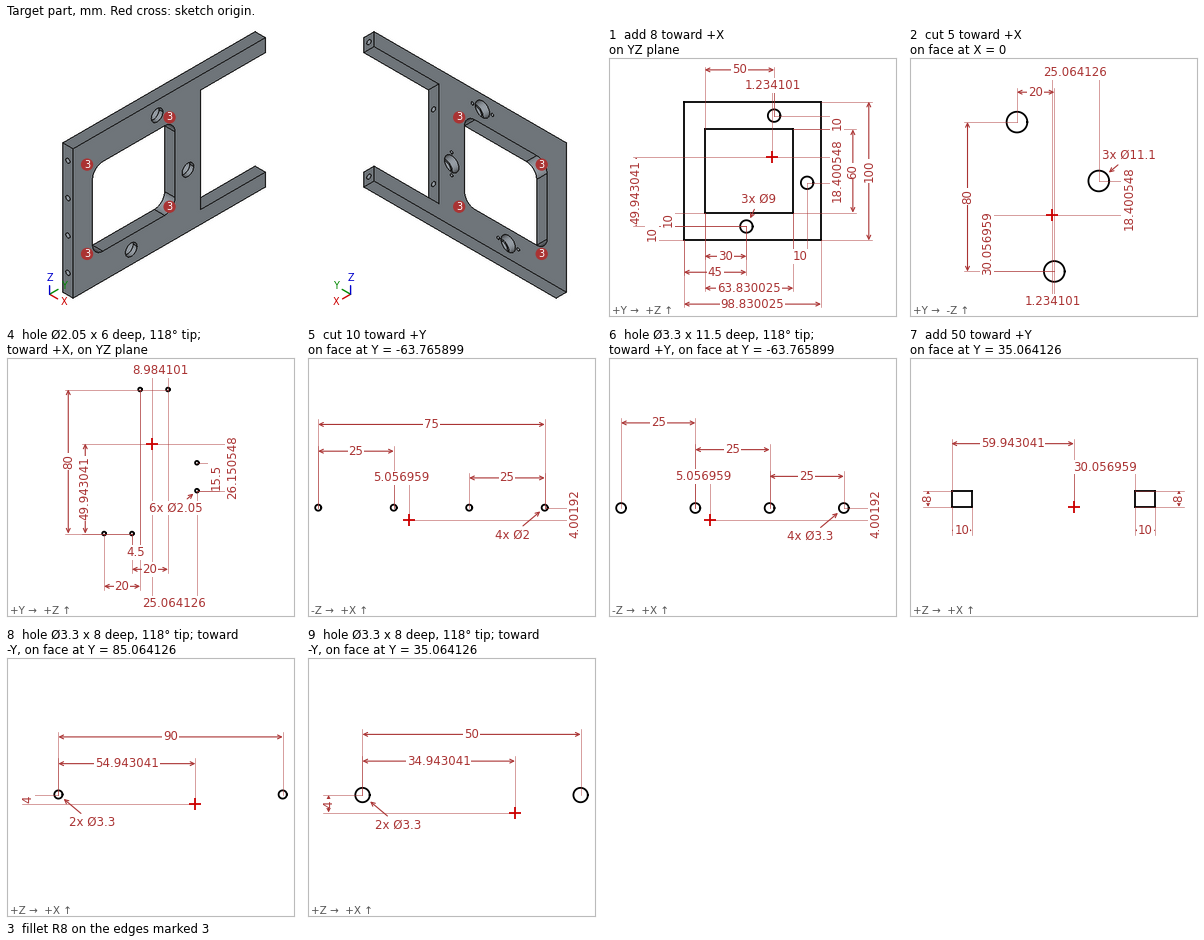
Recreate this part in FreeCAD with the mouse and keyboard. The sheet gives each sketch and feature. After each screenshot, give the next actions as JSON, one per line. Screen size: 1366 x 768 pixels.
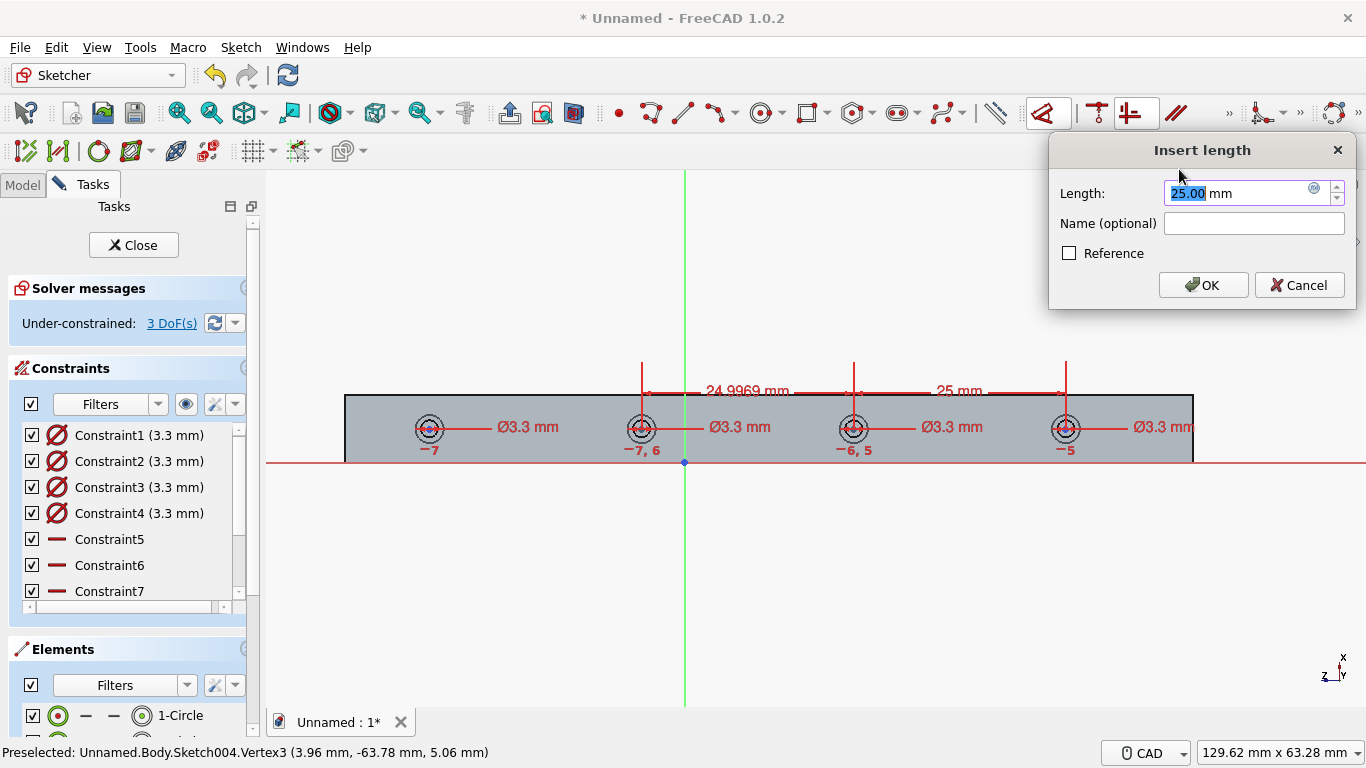
{"action": "type", "text": "25"}
{"action": "key", "text": "Return"}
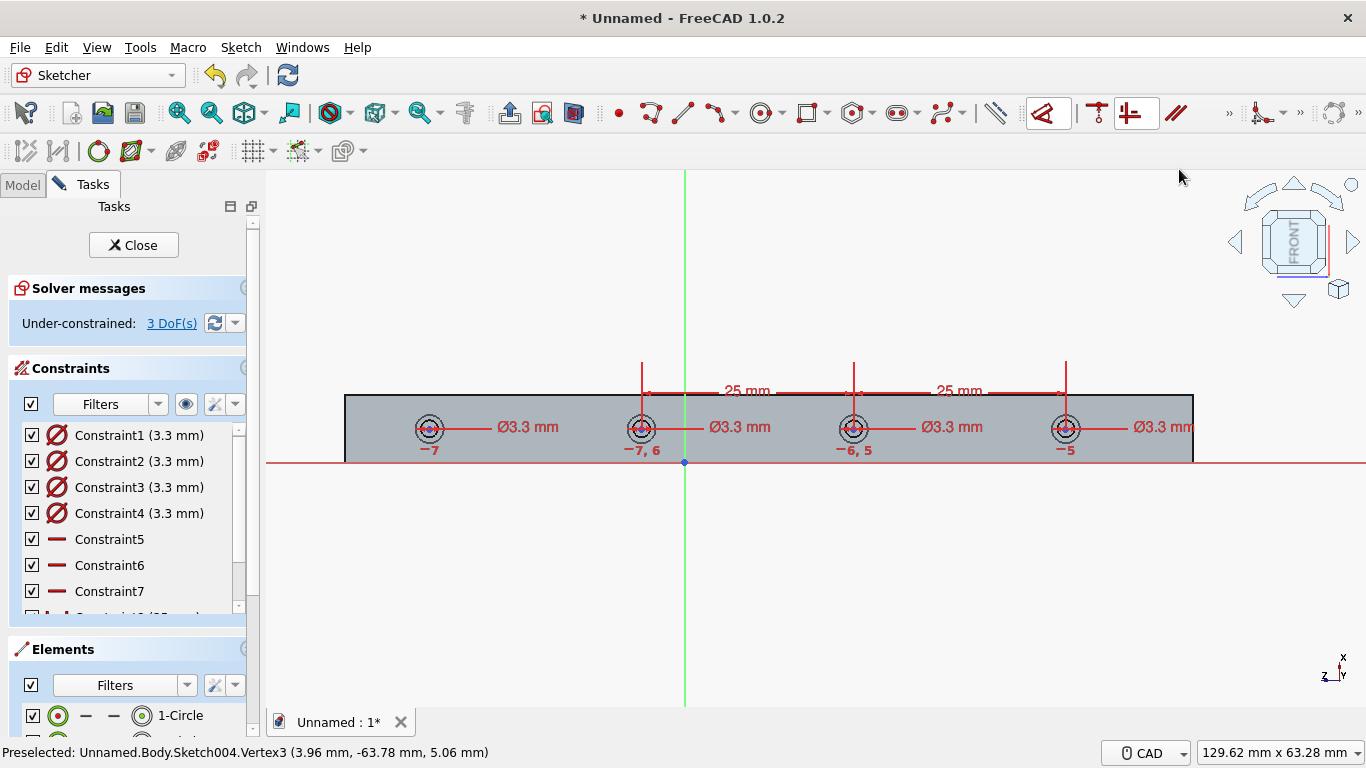
{"action": "left_click", "coordinate": [642, 429]}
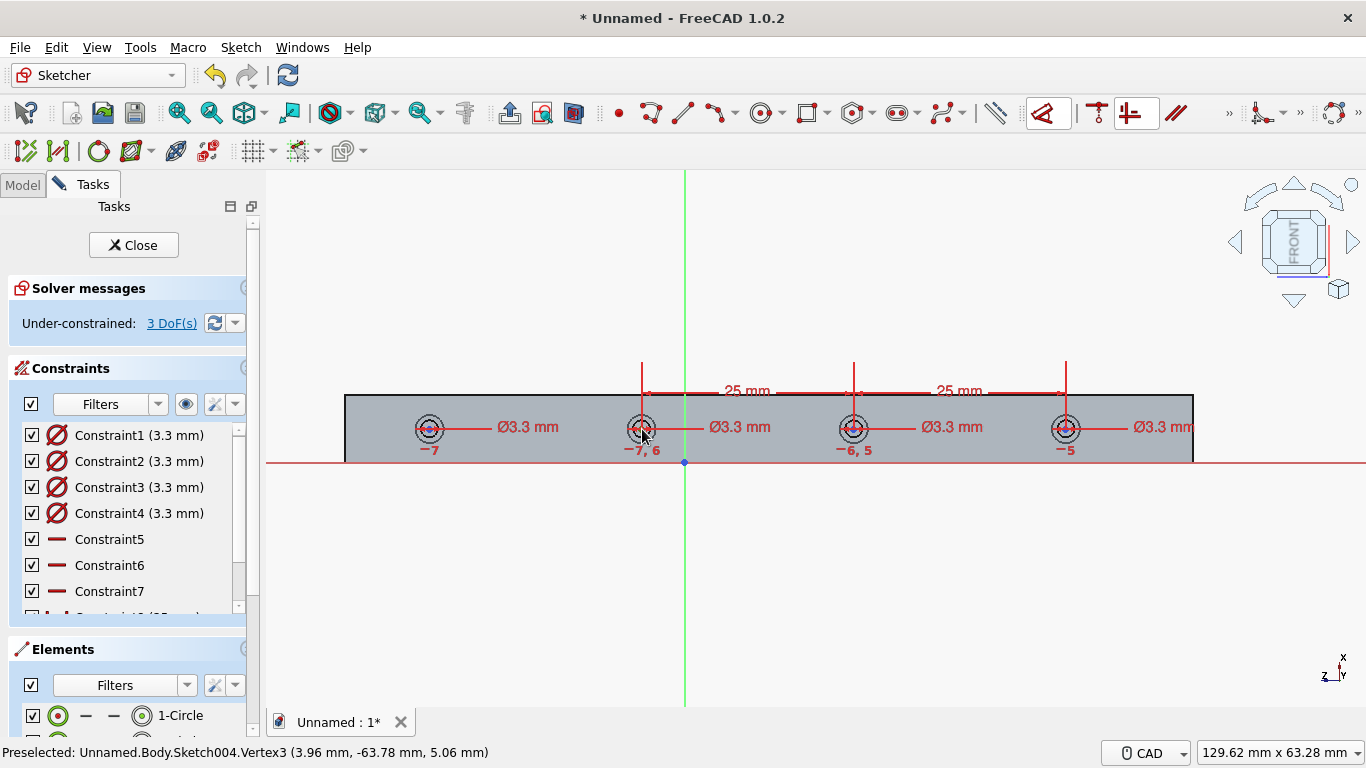
{"action": "left_click", "coordinate": [430, 429]}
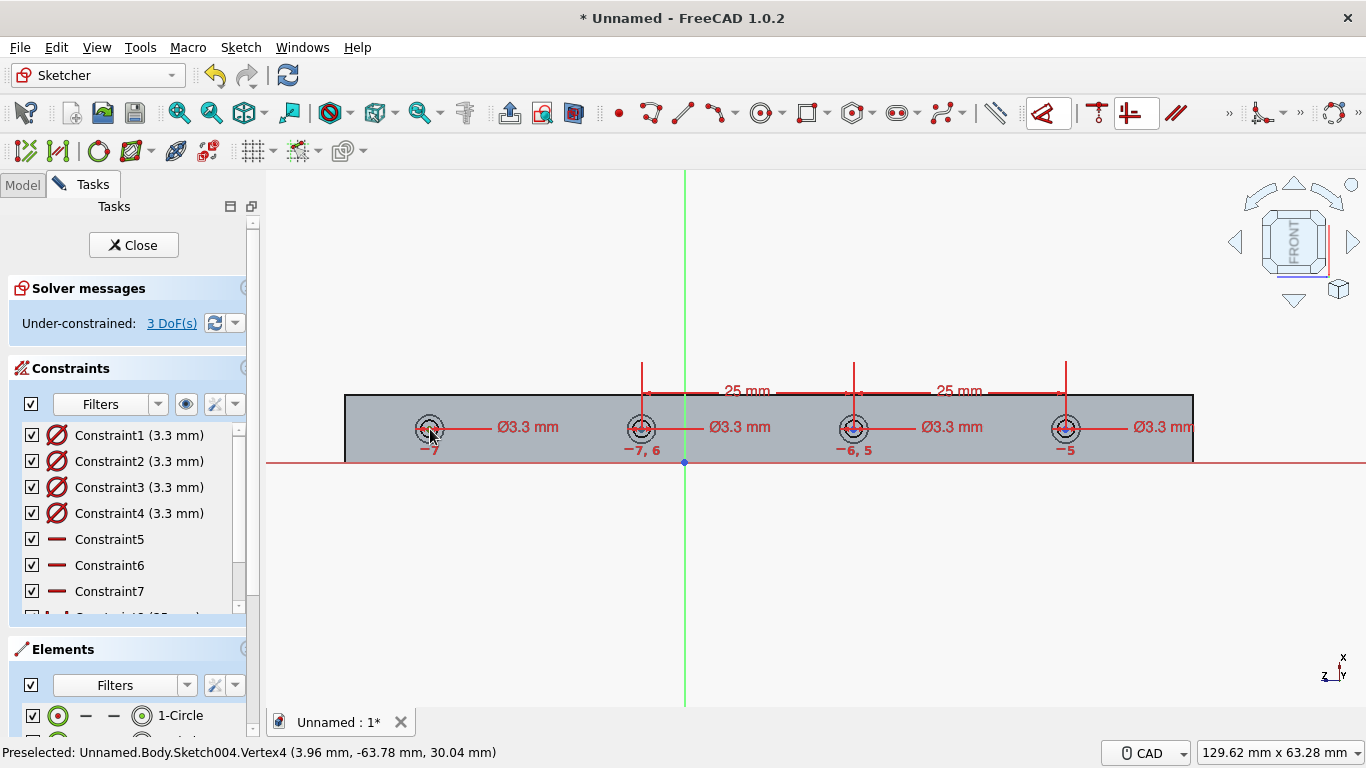
{"action": "key", "text": "l"}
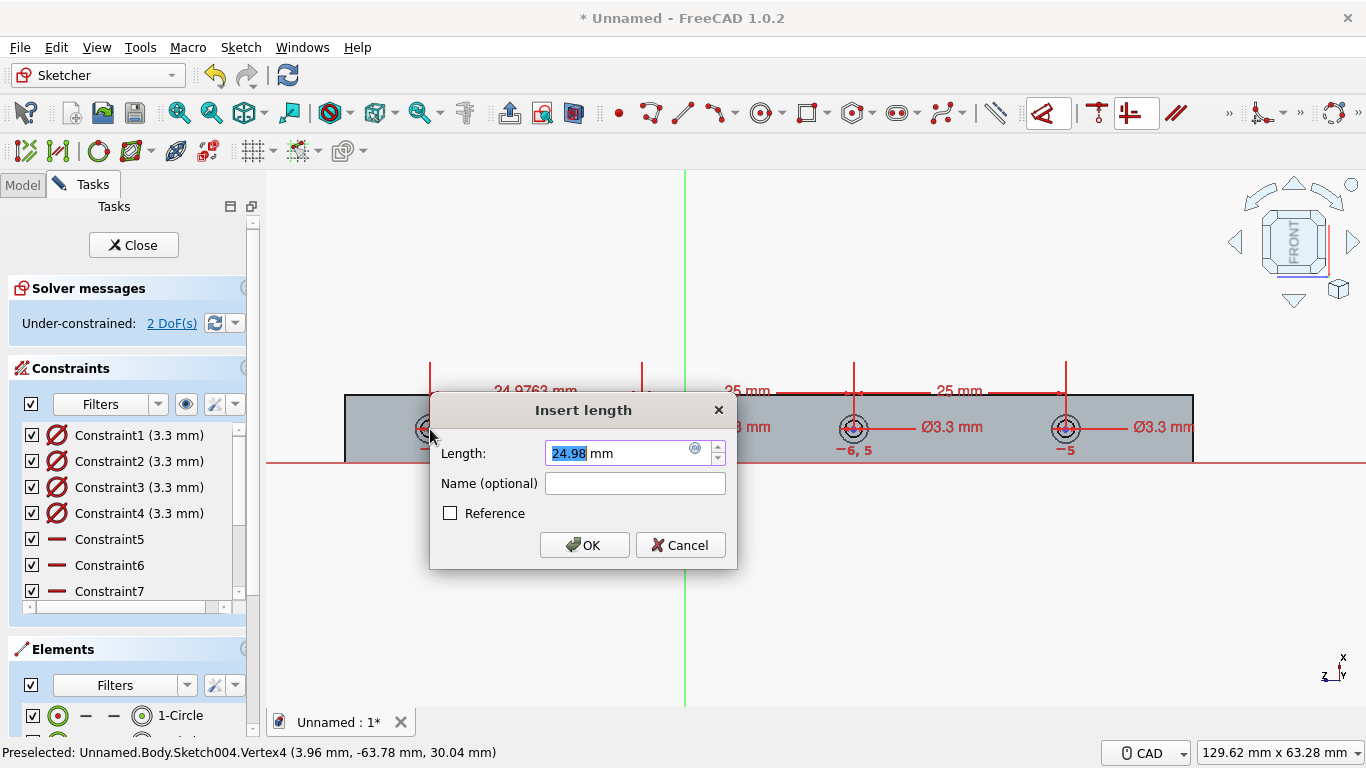
{"action": "type", "text": "25"}
{"action": "key", "text": "Return"}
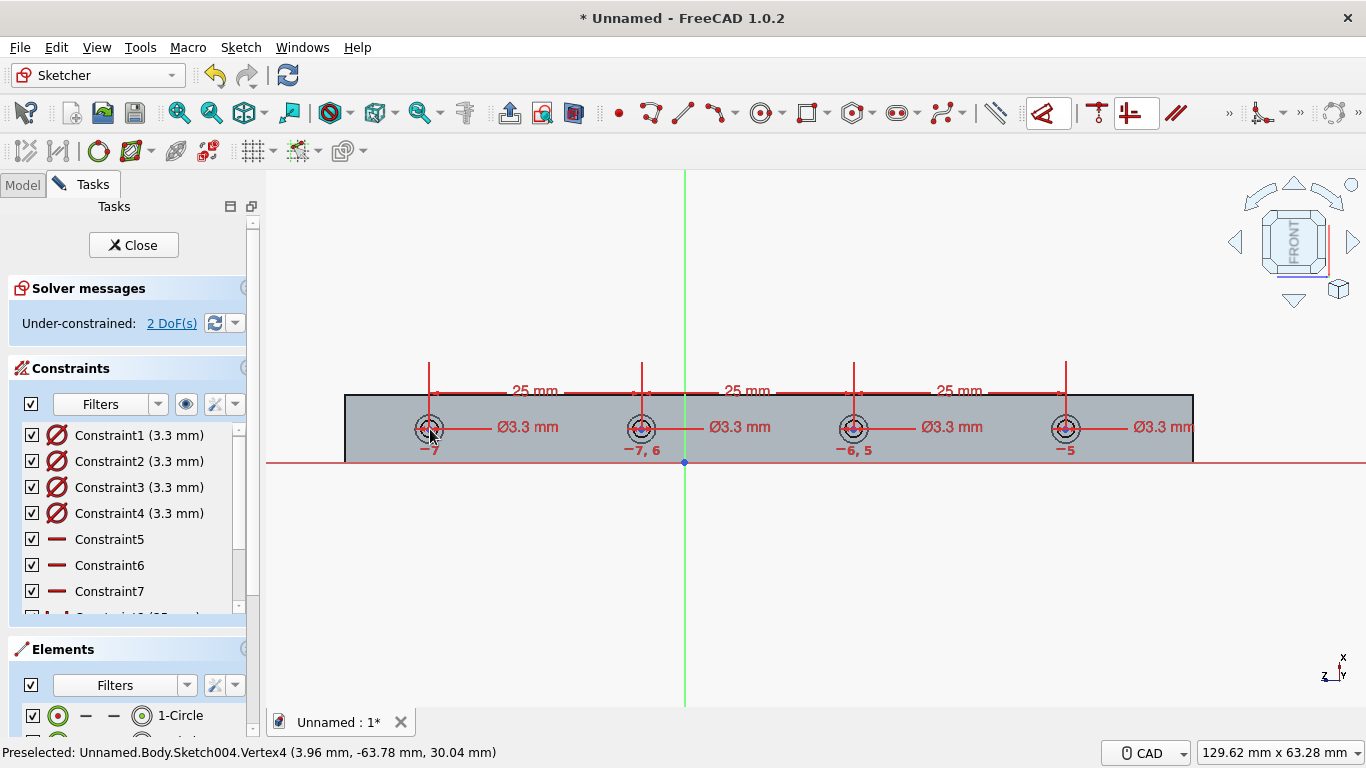
{"action": "left_click", "coordinate": [1066, 429]}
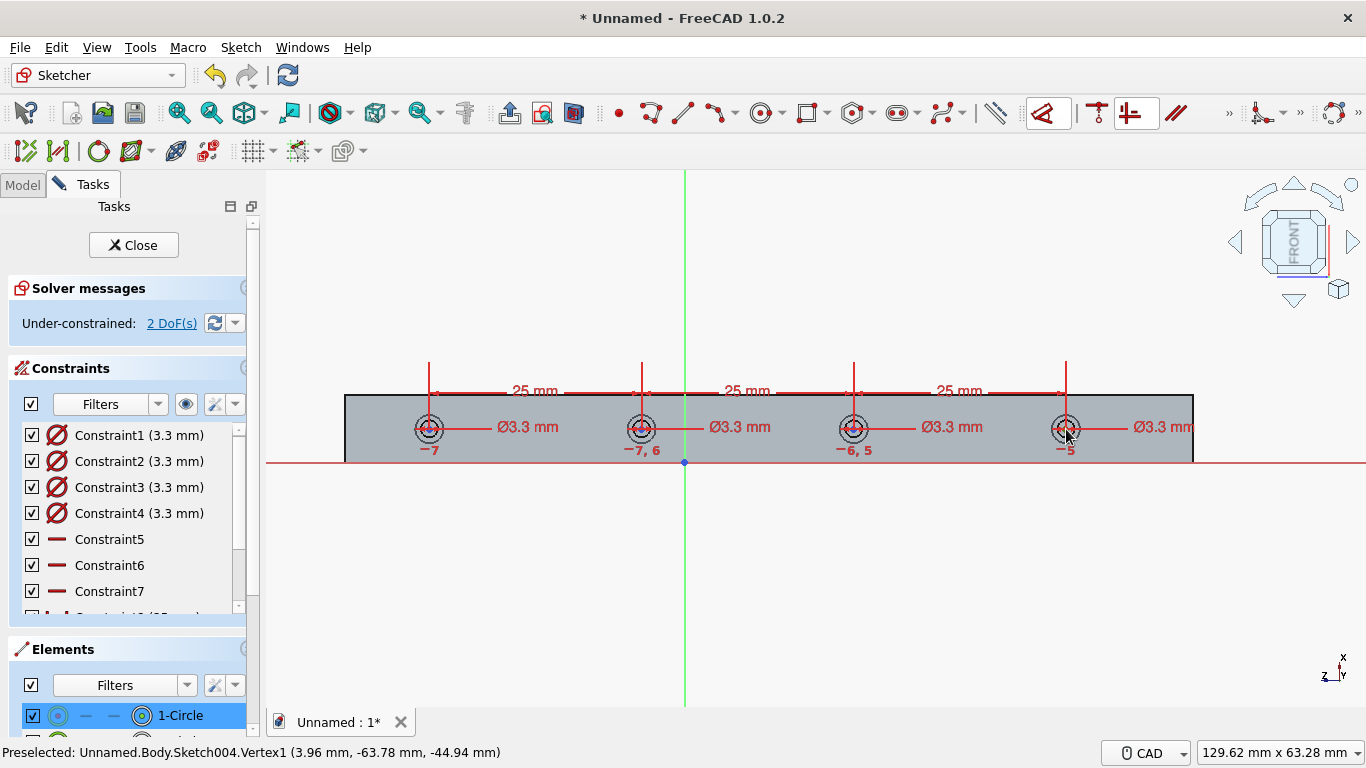
{"action": "key", "text": "i"}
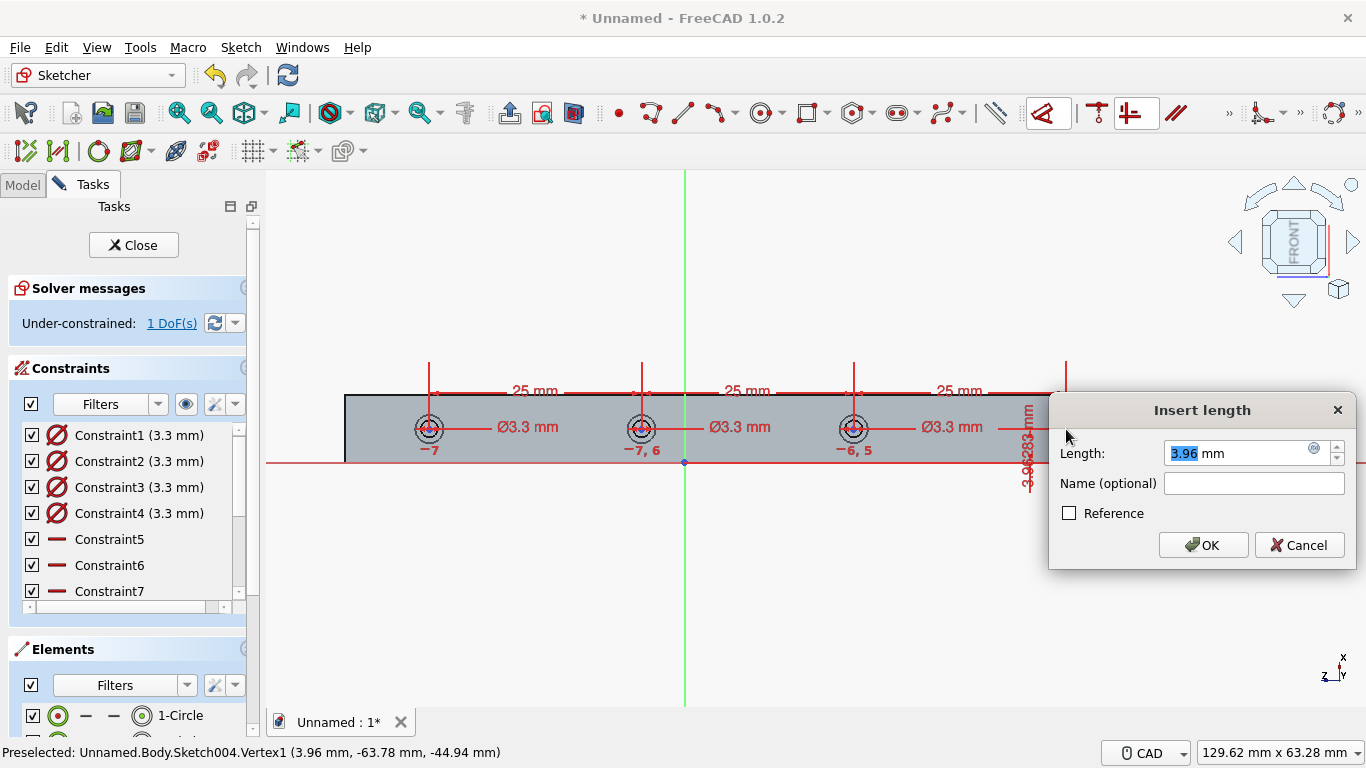
{"action": "type", "text": "4.00192"}
{"action": "key", "text": "Return"}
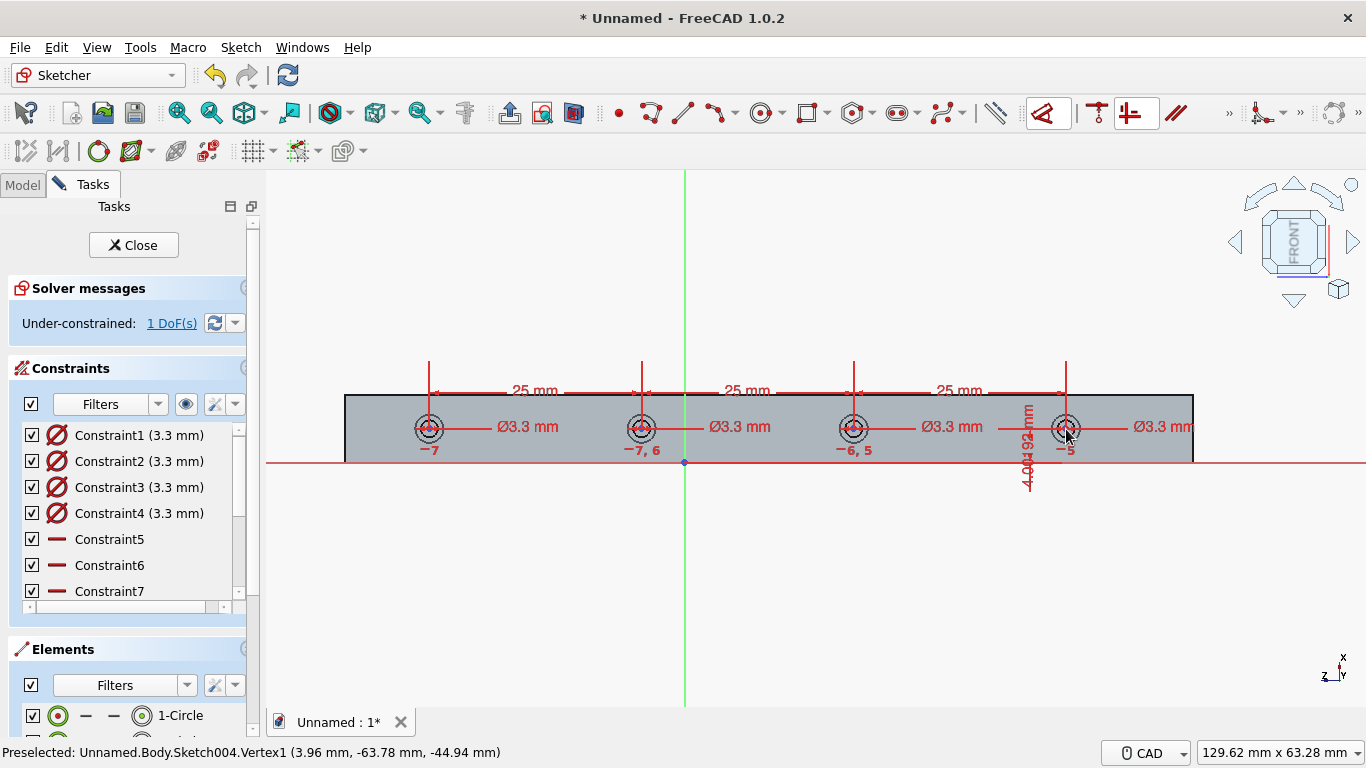
{"action": "left_click", "coordinate": [642, 429]}